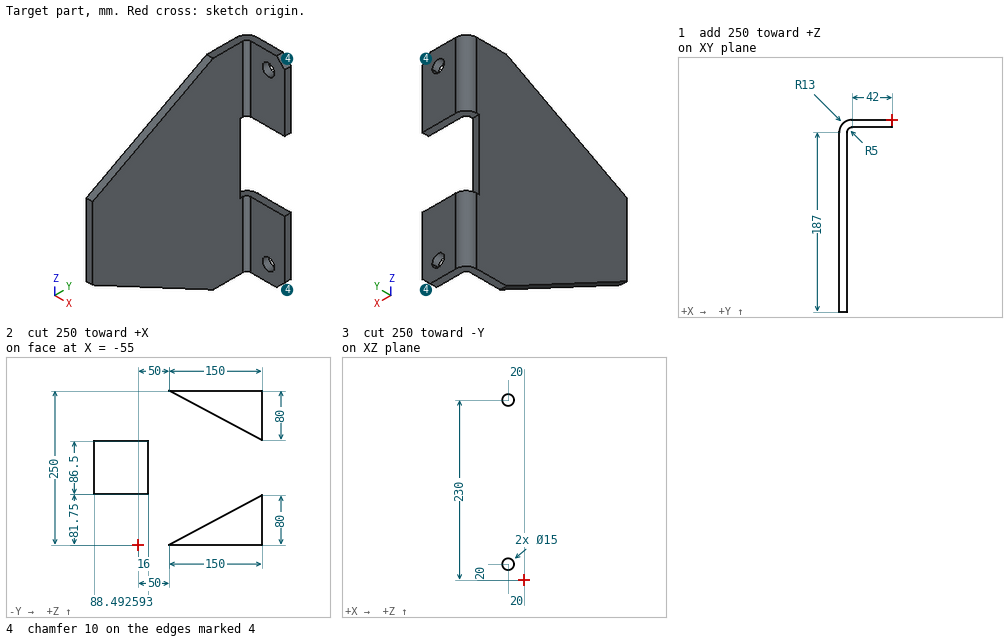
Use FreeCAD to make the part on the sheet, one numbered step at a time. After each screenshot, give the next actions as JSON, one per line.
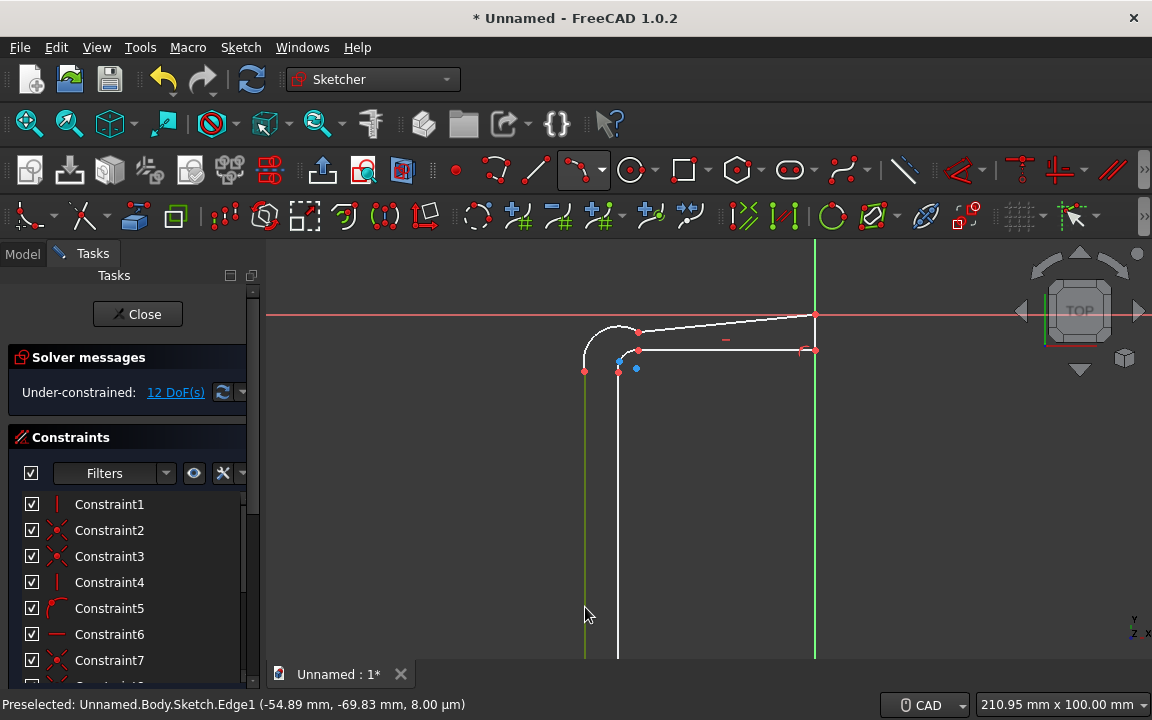
{"action": "left_click", "coordinate": [614, 327]}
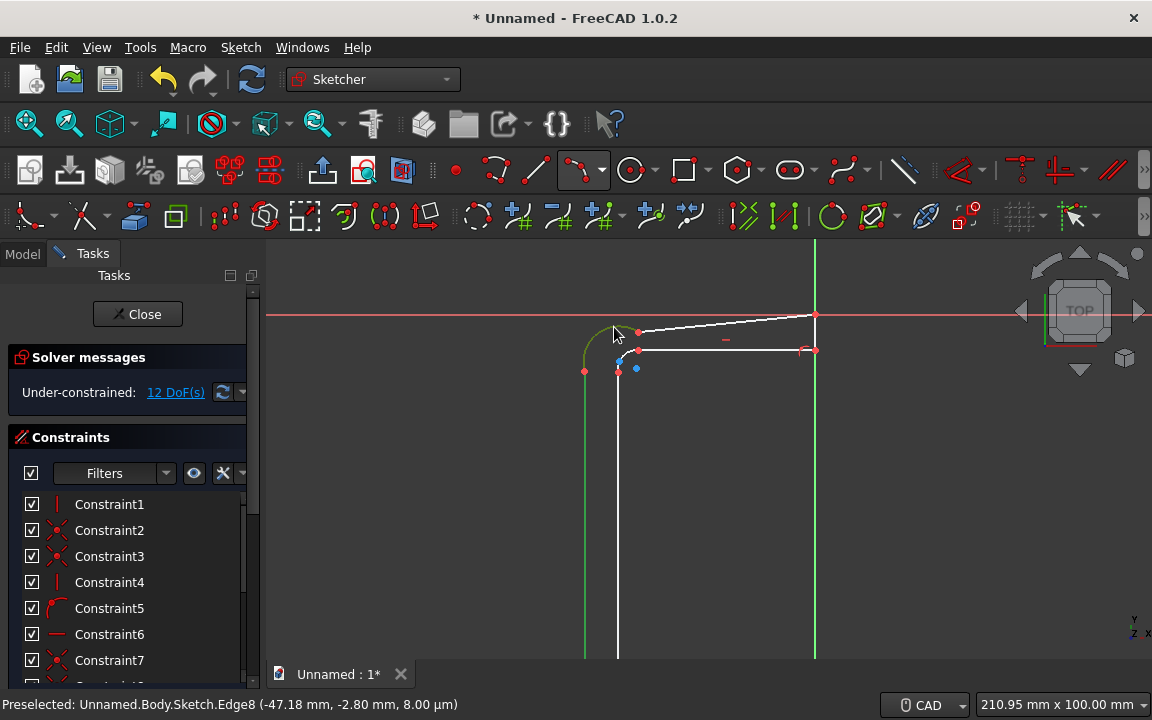
{"action": "key", "text": "t"}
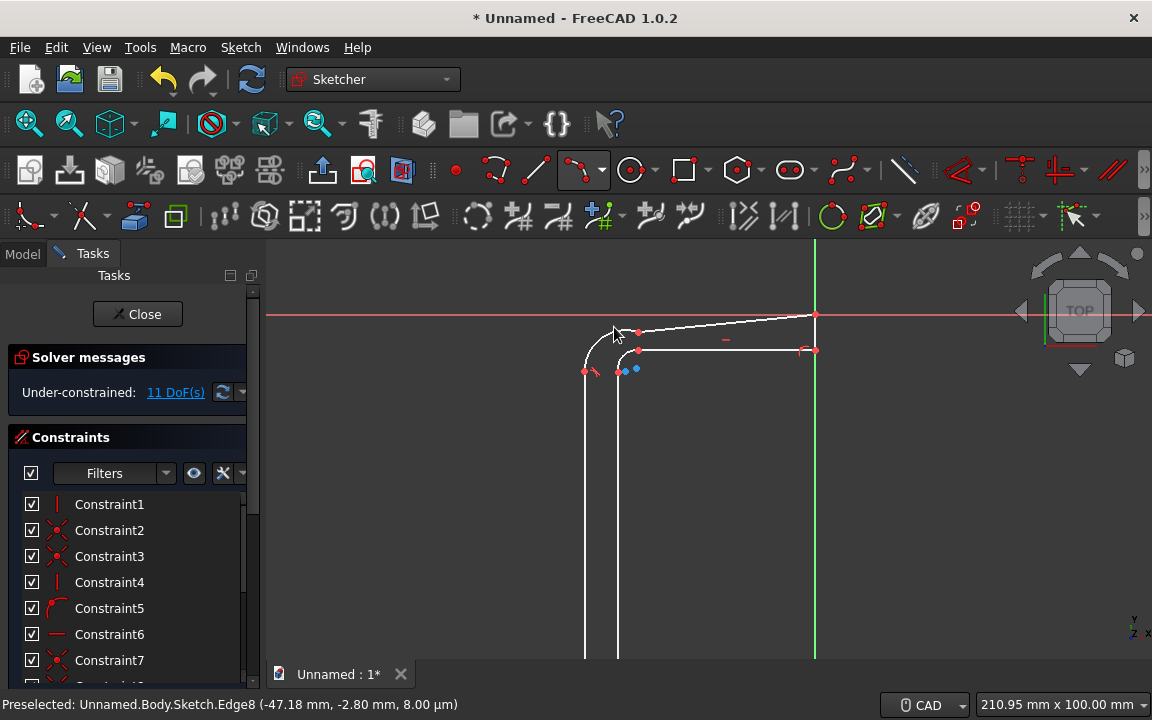
{"action": "left_click", "coordinate": [618, 607]}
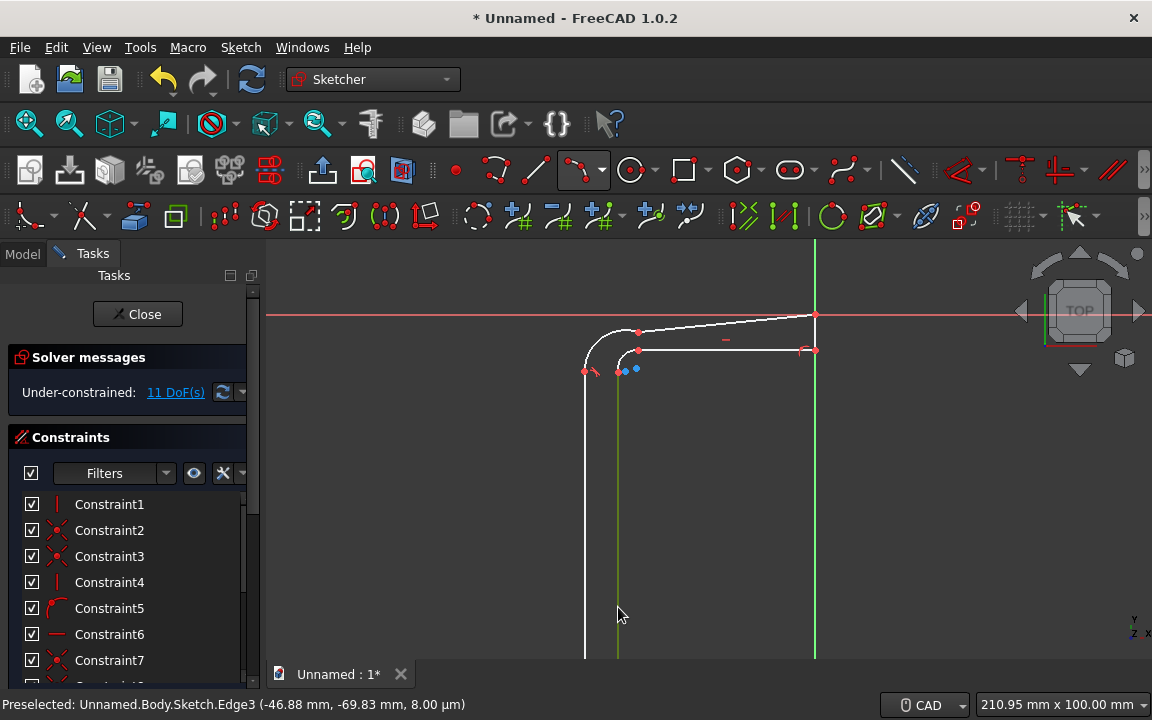
{"action": "scroll", "coordinate": [628, 352], "scroll_direction": "up", "scroll_amount": 2}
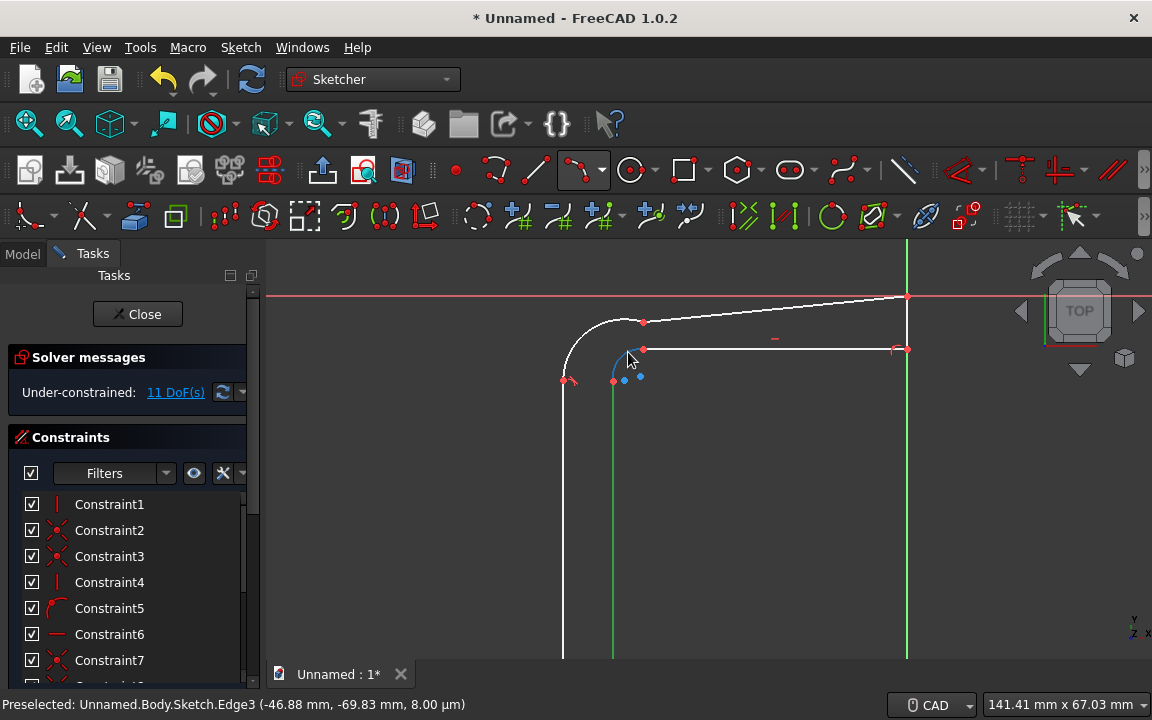
{"action": "left_click", "coordinate": [628, 352]}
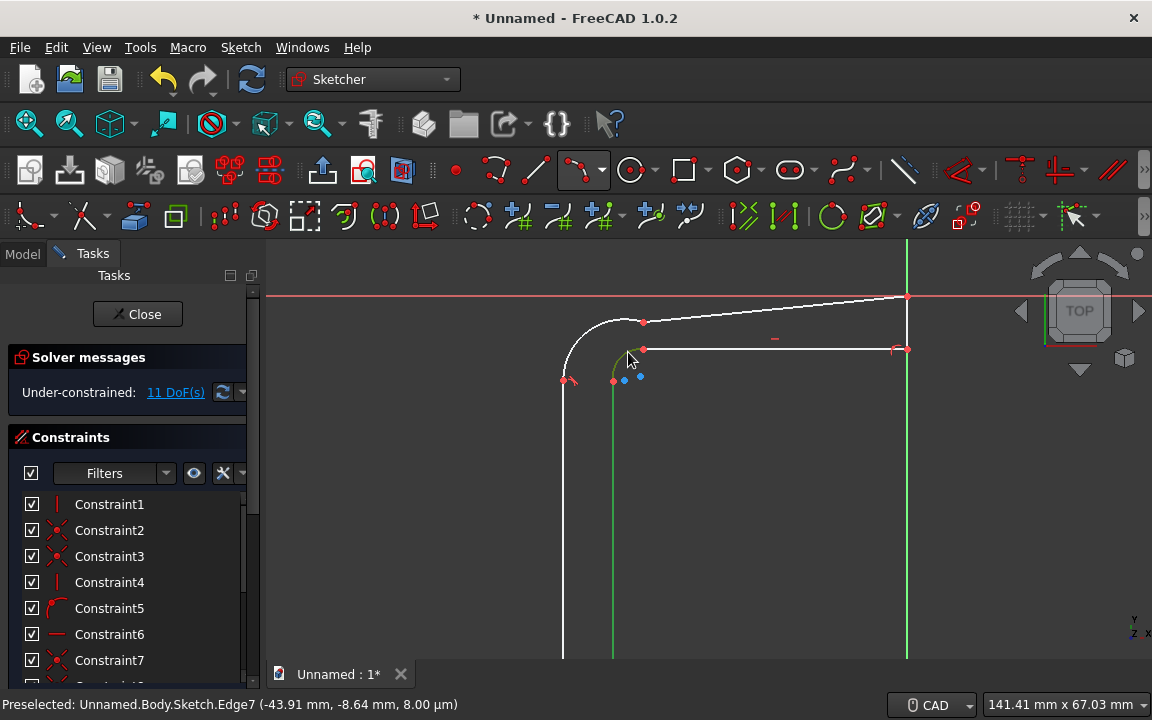
{"action": "key", "text": "t"}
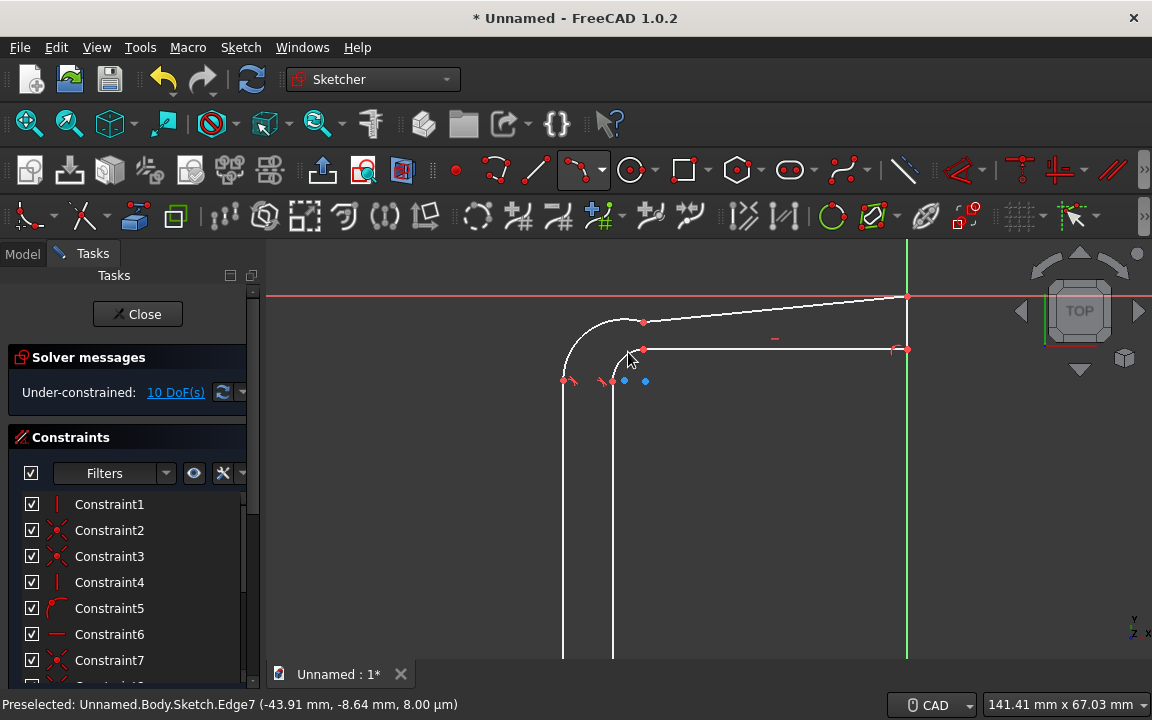
{"action": "left_click", "coordinate": [722, 349]}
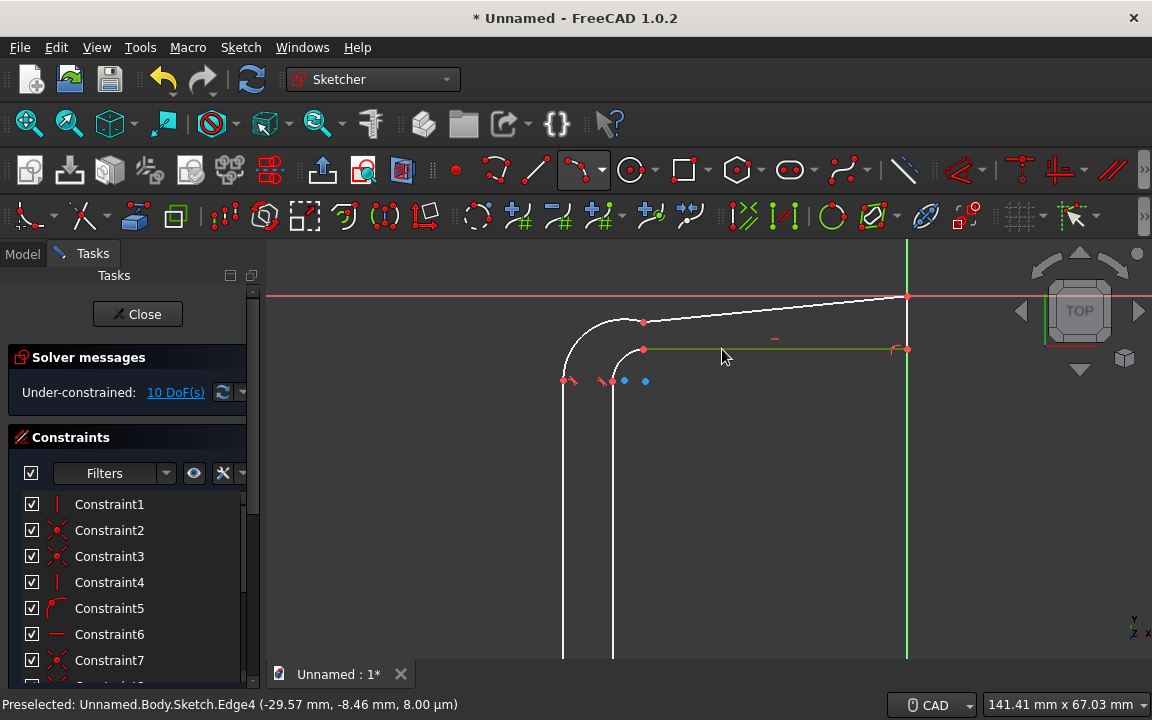
{"action": "left_click", "coordinate": [629, 353]}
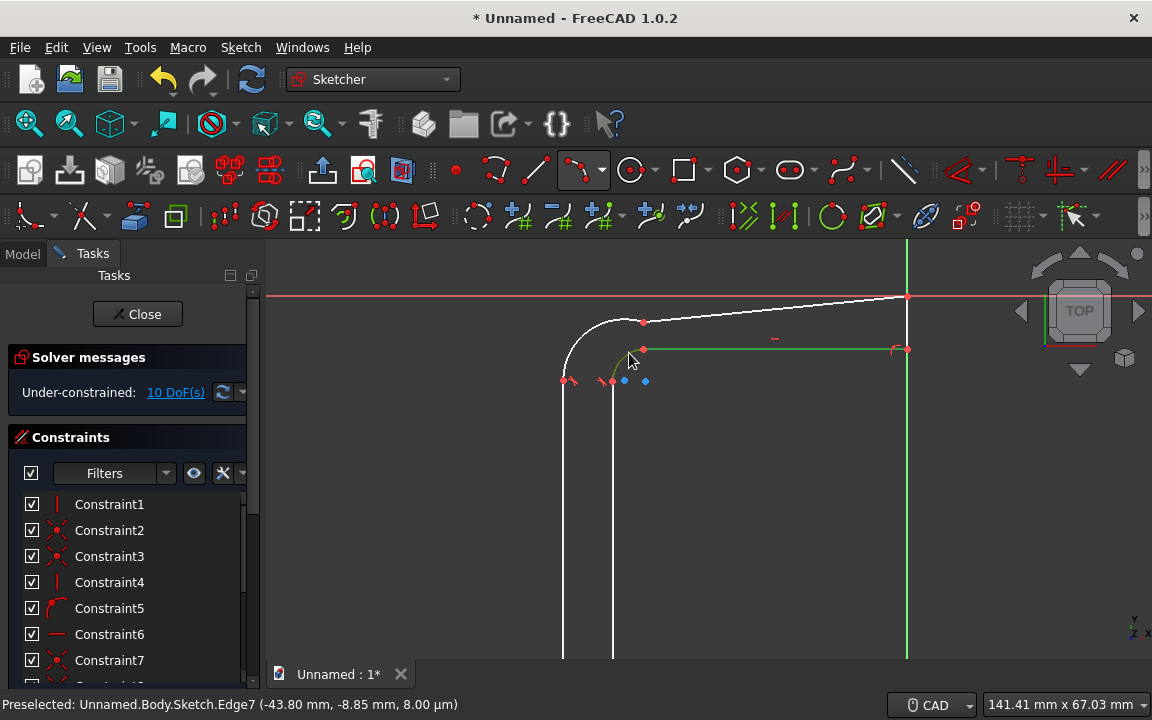
{"action": "key", "text": "t"}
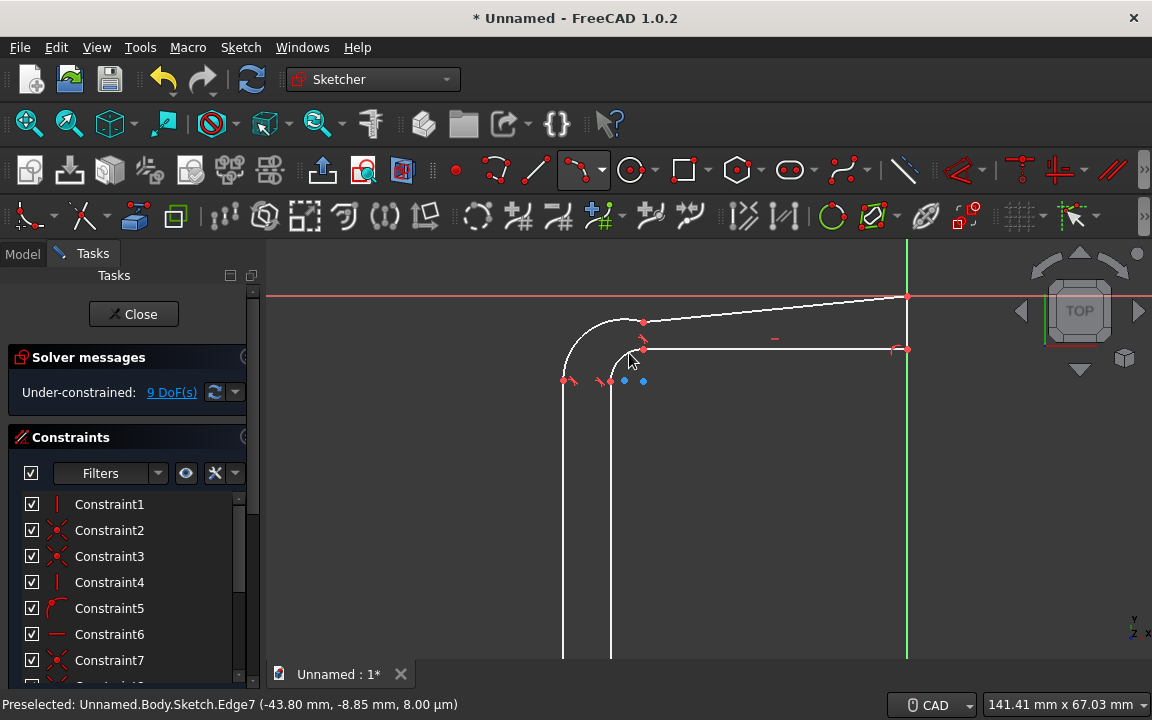
{"action": "left_click", "coordinate": [722, 314]}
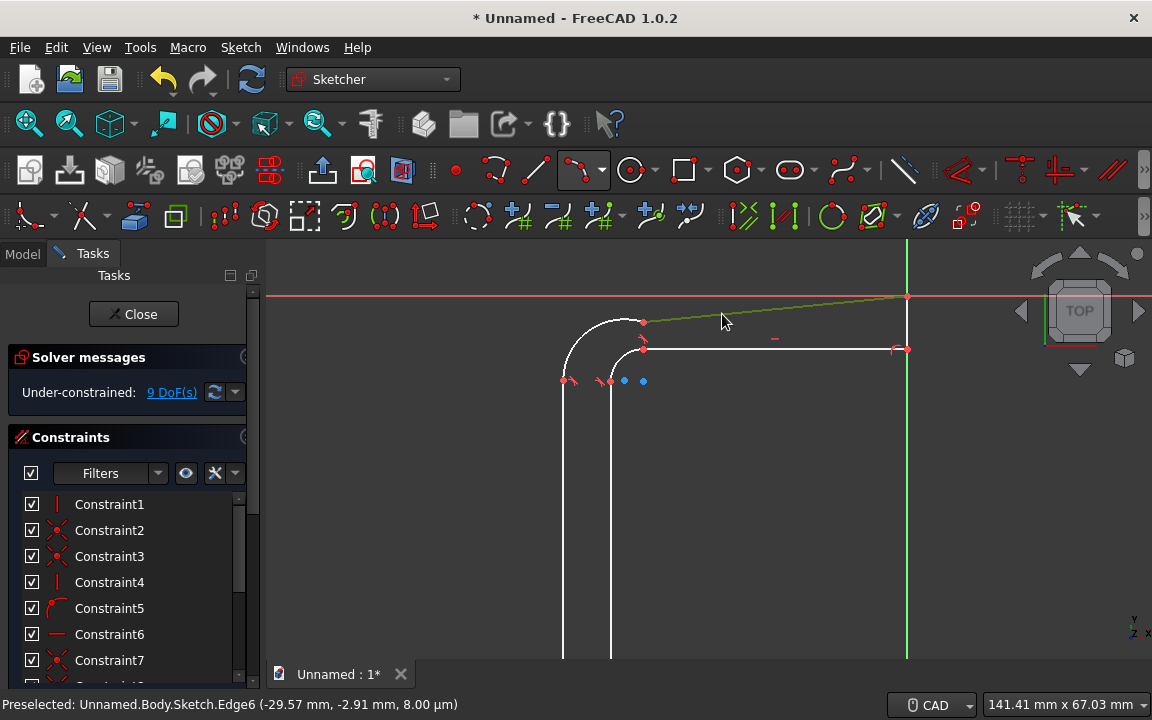
{"action": "left_click", "coordinate": [609, 321]}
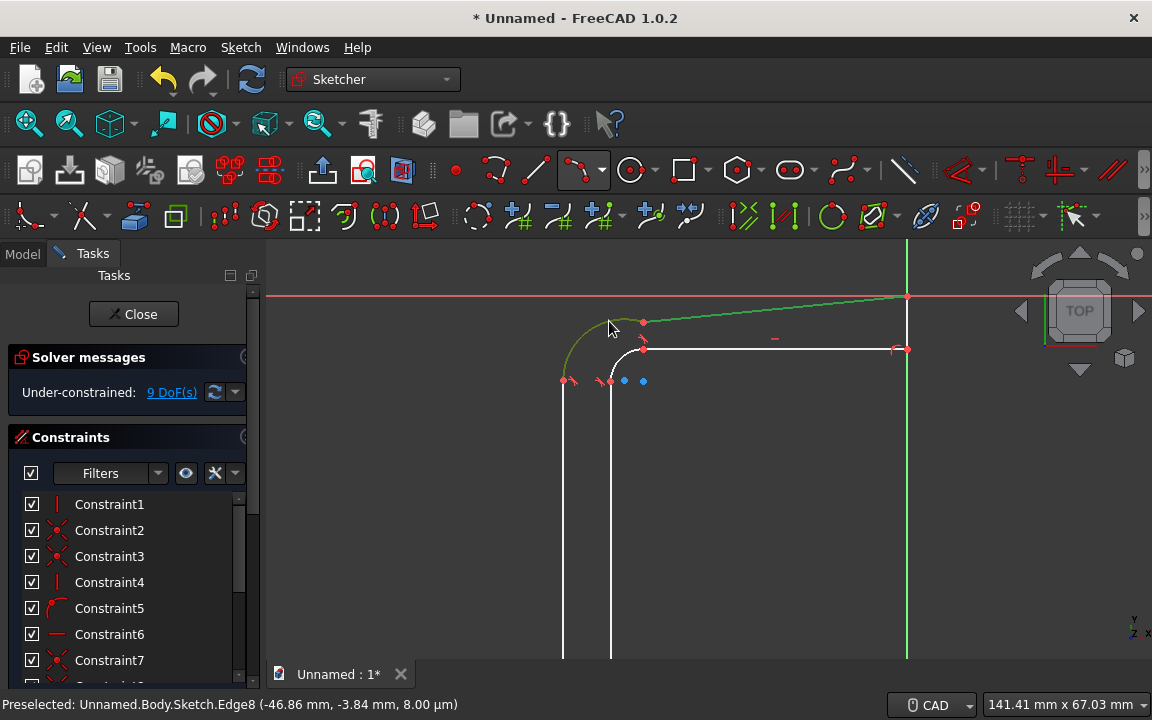
{"action": "key", "text": "t"}